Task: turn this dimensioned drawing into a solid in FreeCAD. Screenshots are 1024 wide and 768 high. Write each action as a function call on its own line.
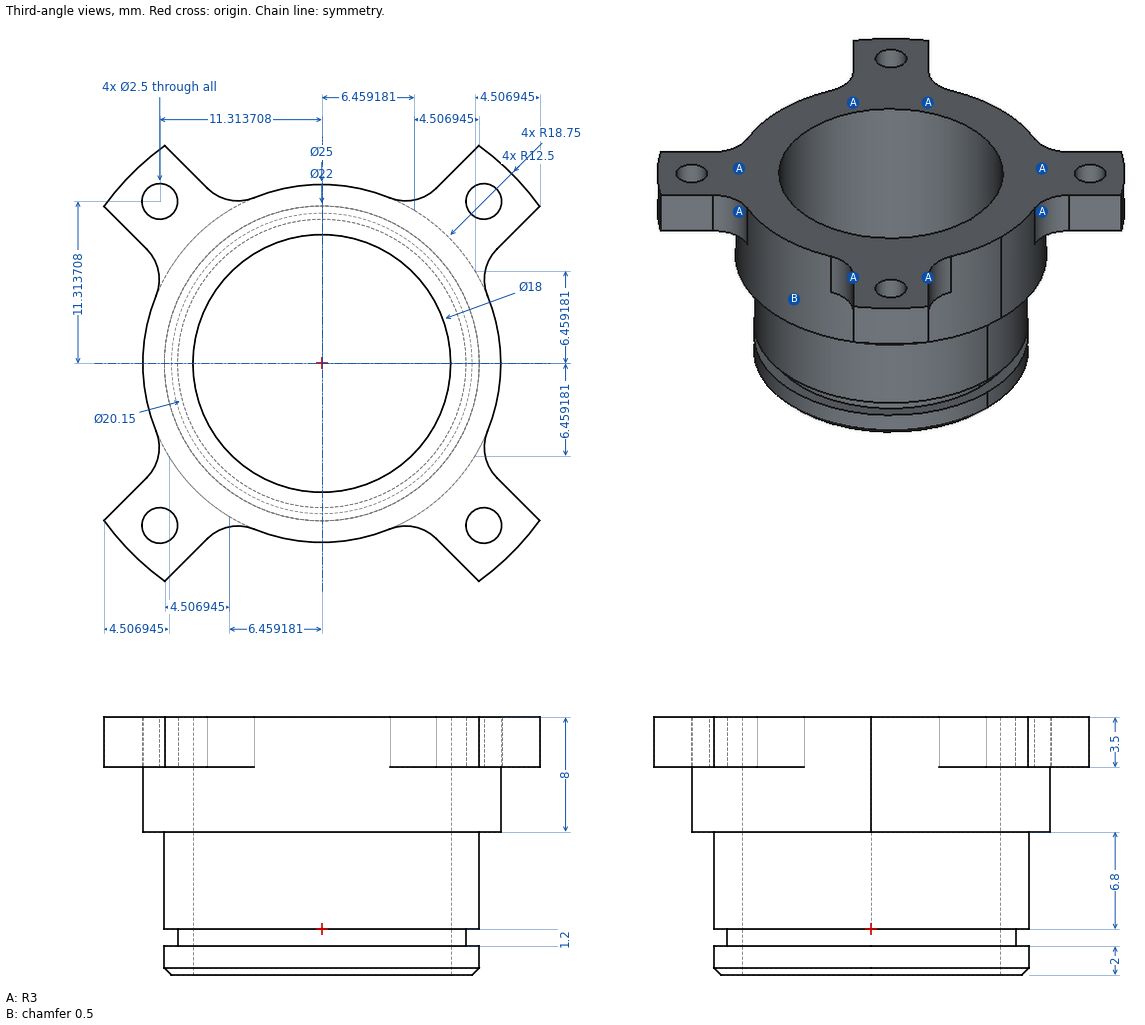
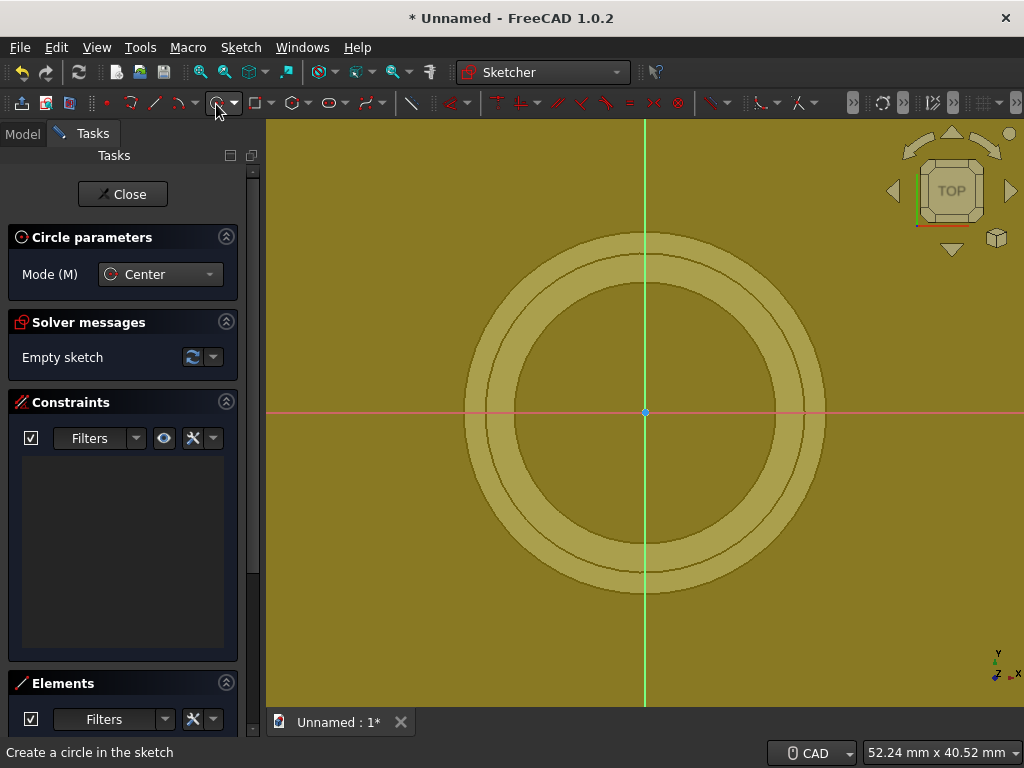
click(645, 413)
click(773, 285)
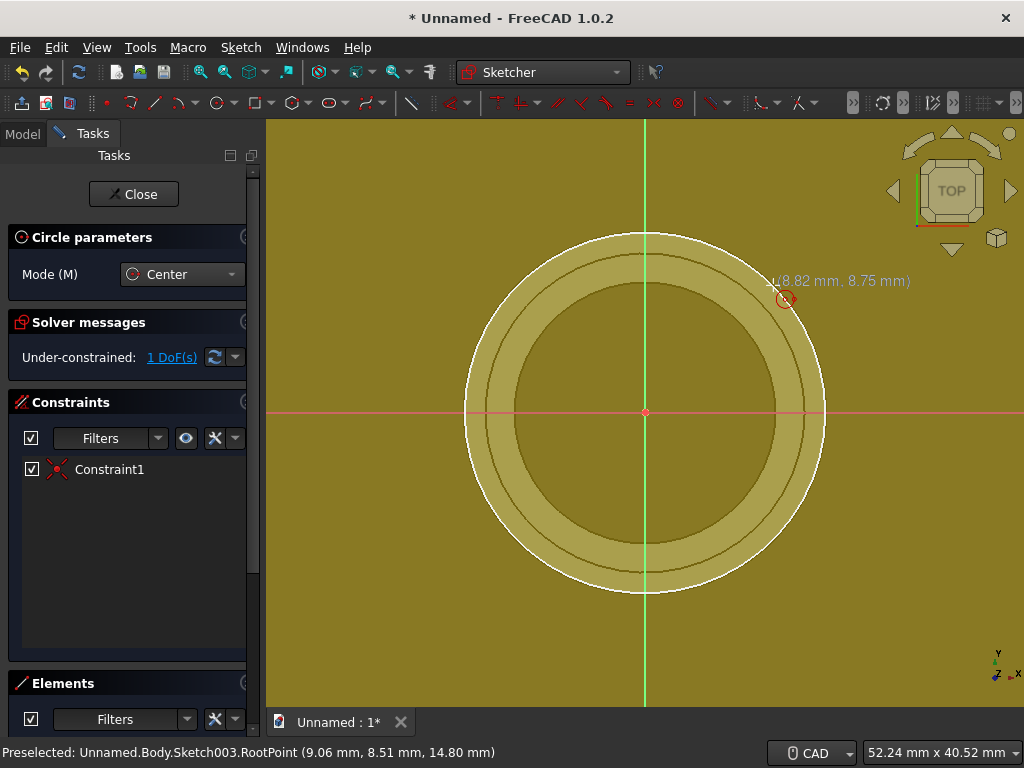
click(645, 413)
click(737, 321)
key(Escape)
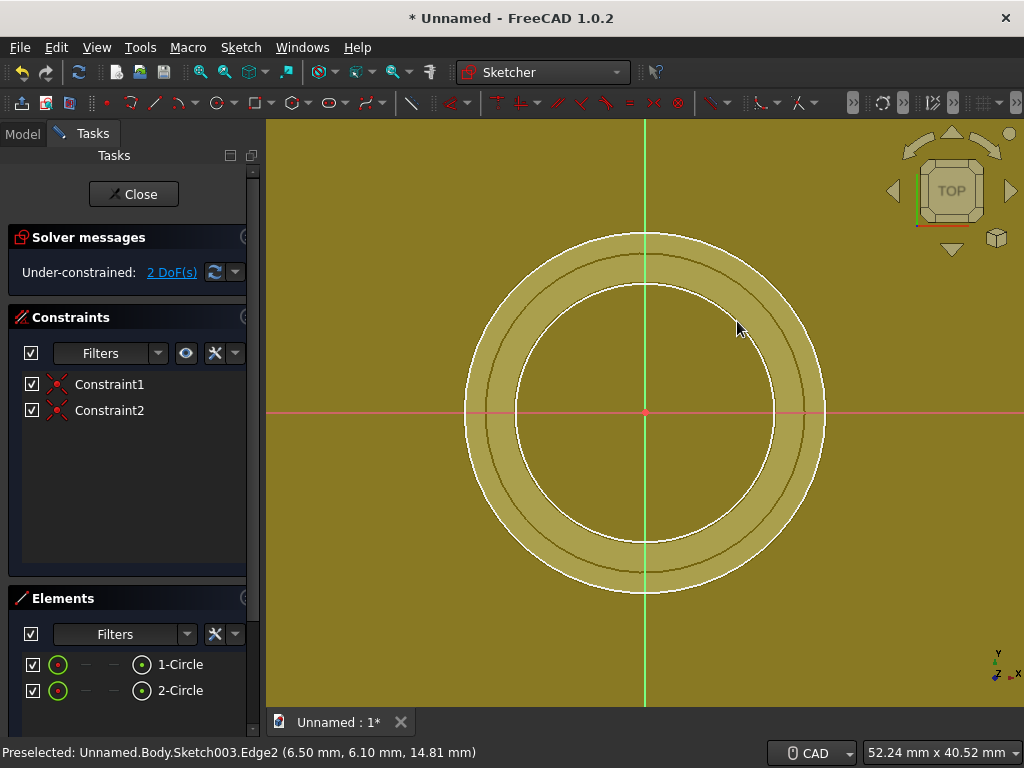
click(450, 104)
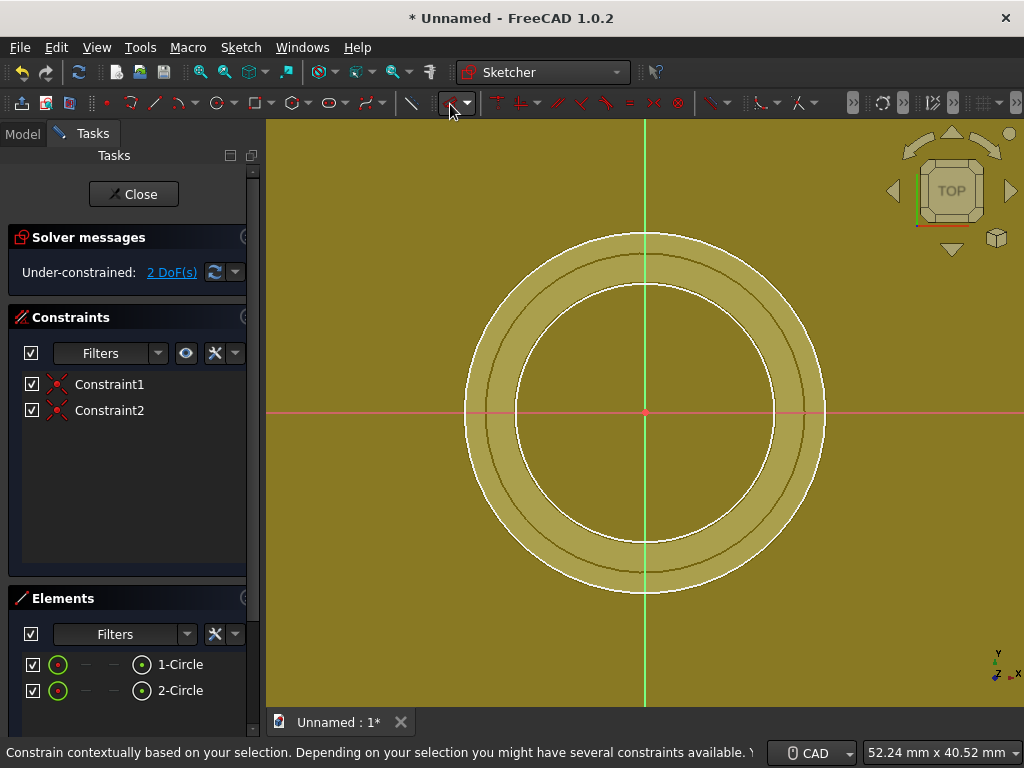
click(772, 285)
click(795, 262)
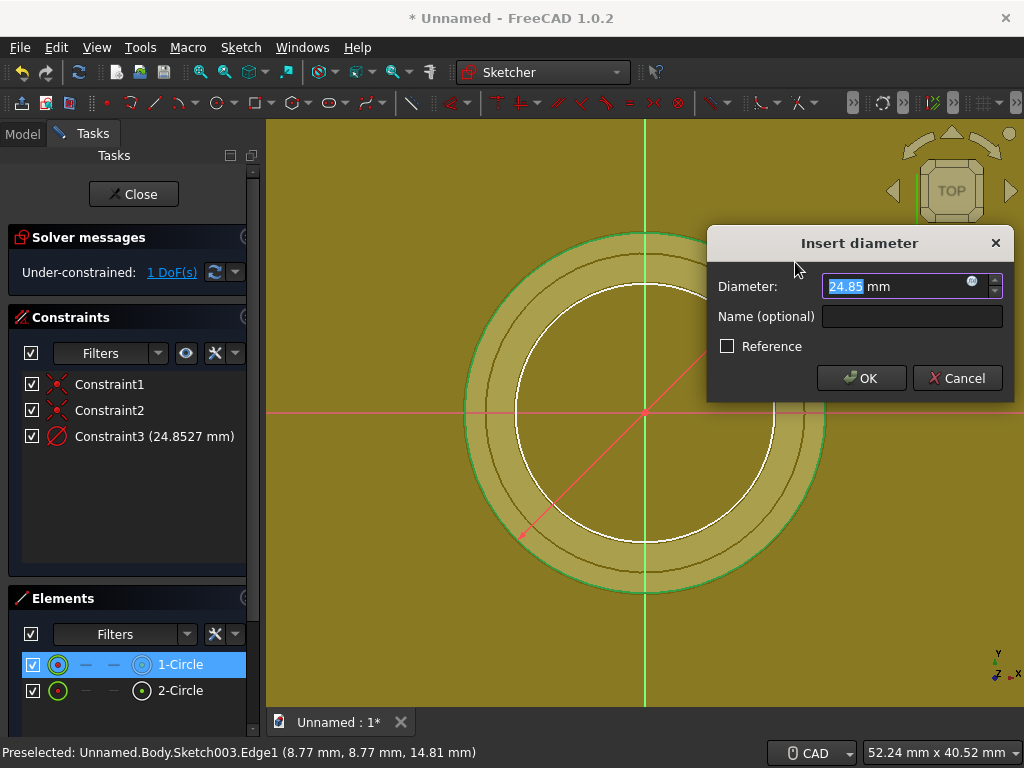
text(25)
key(Return)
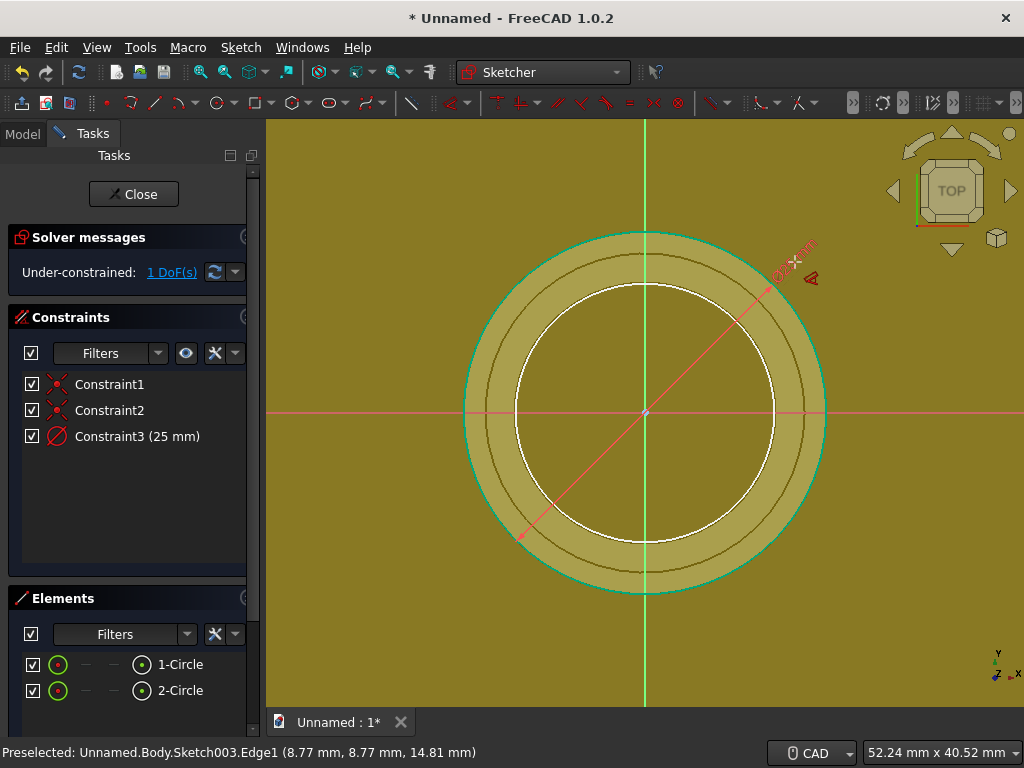
click(736, 321)
click(759, 298)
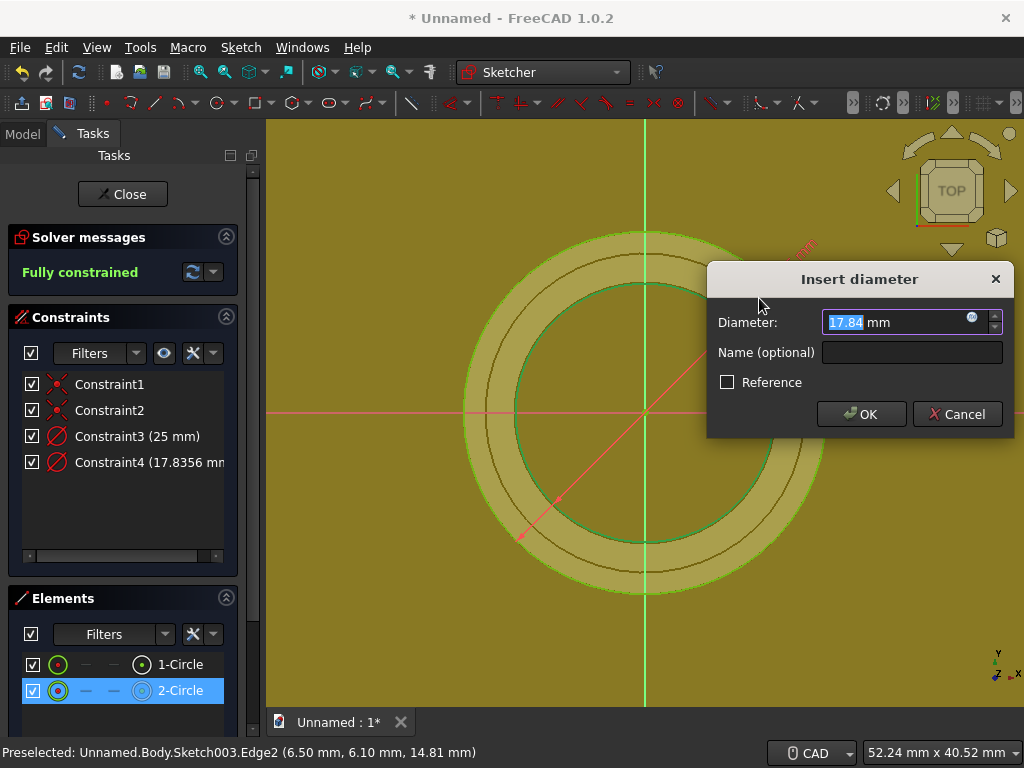
text(18)
key(Return)
key(Escape)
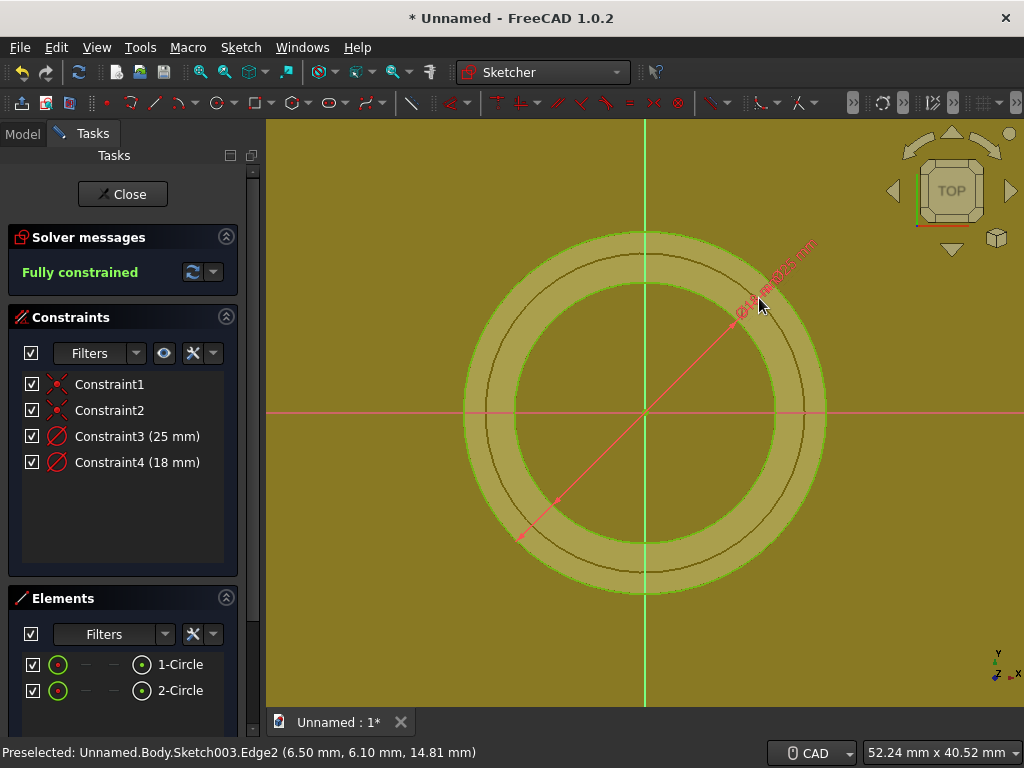
click(123, 194)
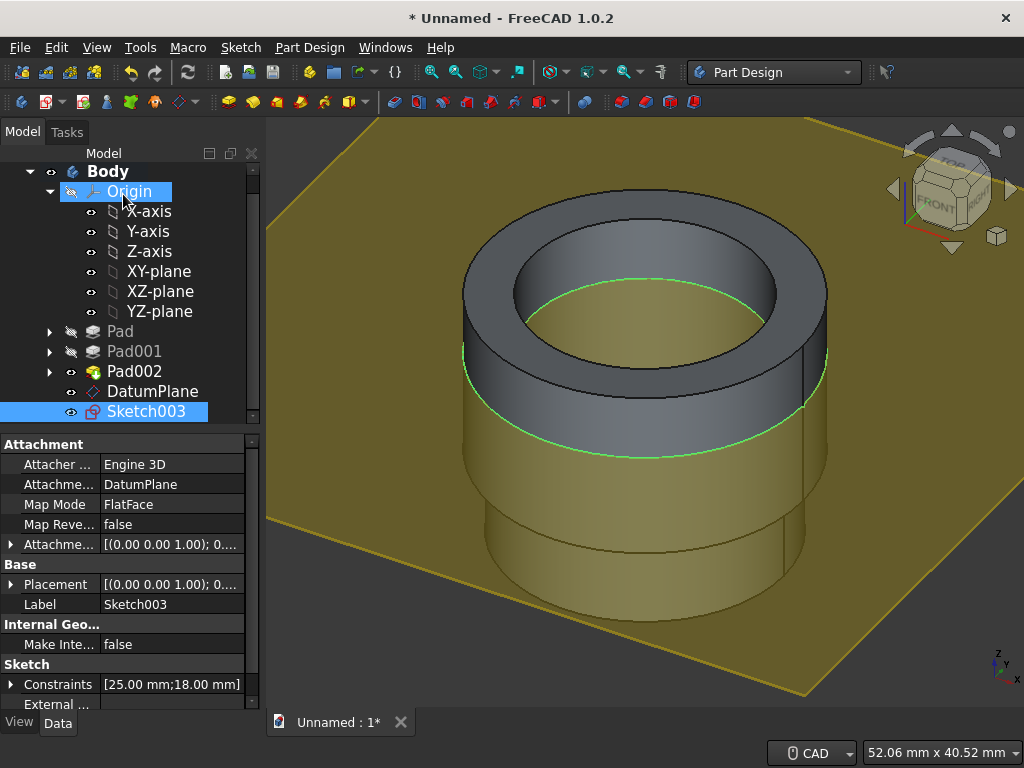
click(396, 102)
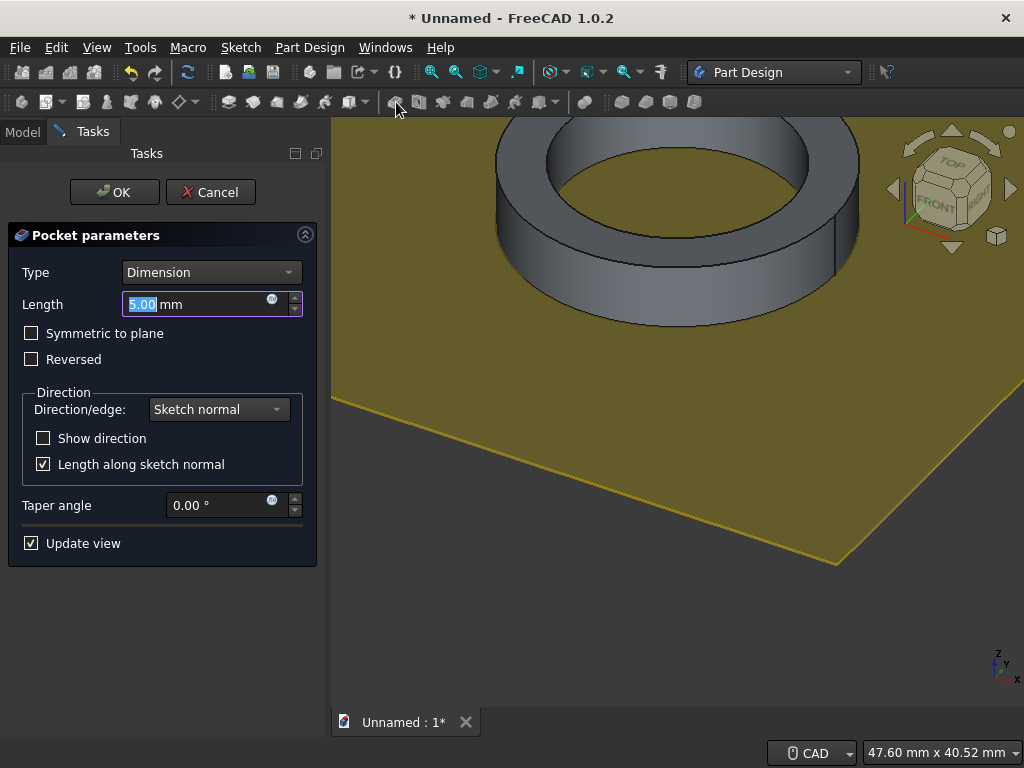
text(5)
key(Tab)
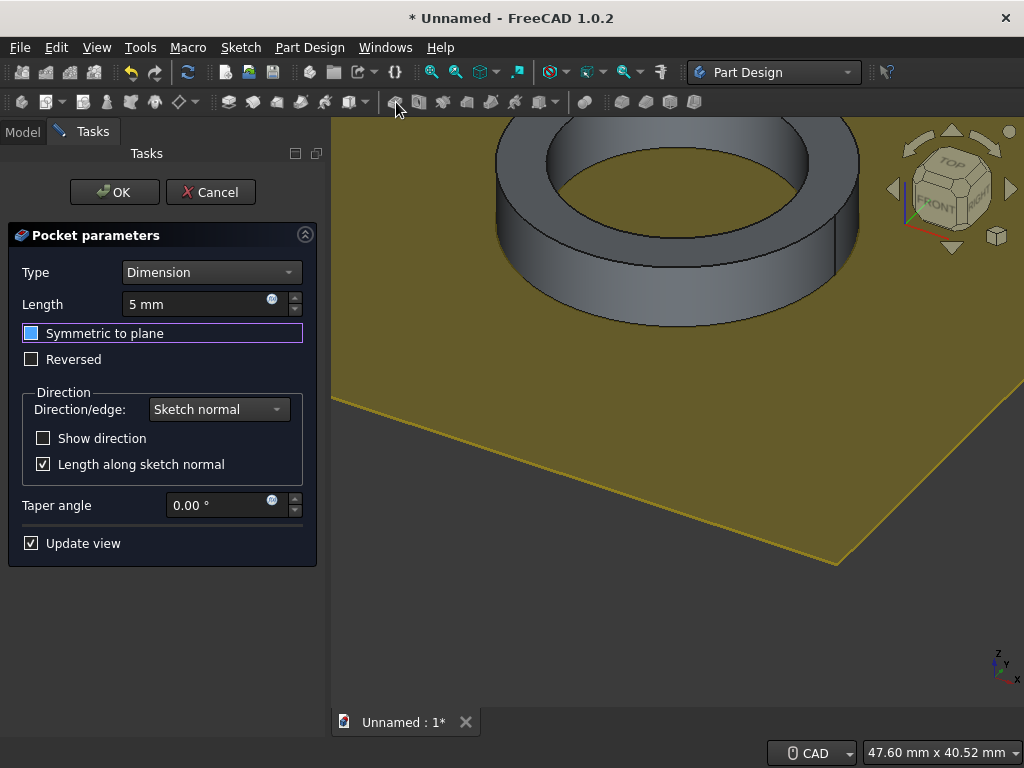
click(30, 359)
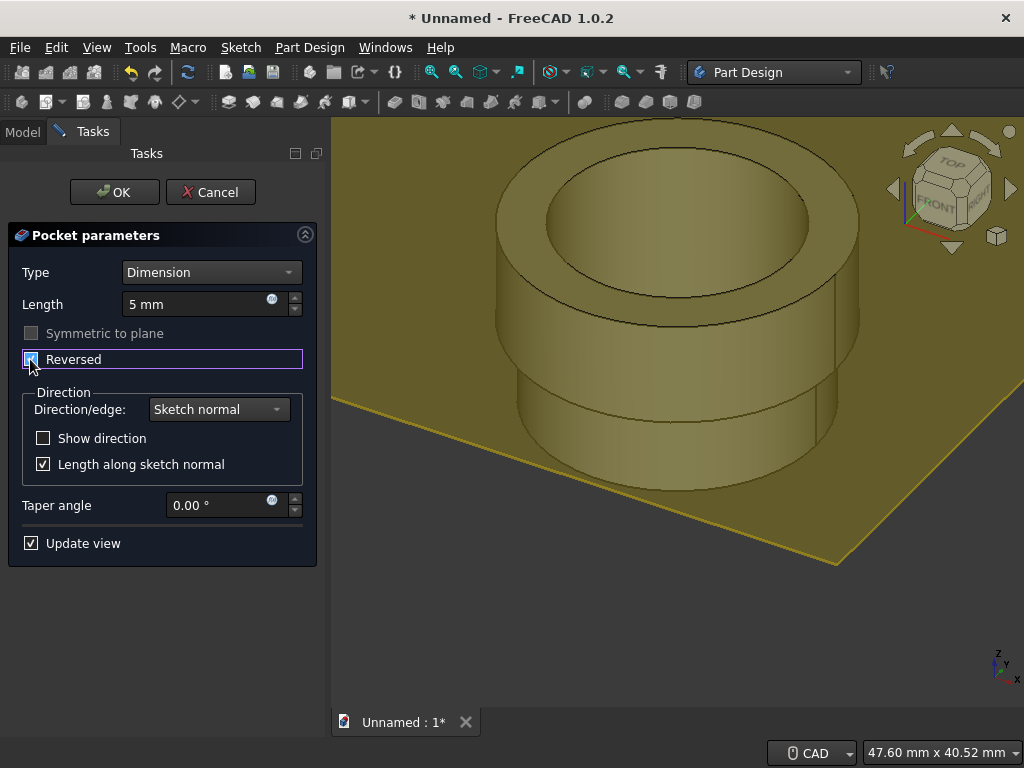
click(115, 192)